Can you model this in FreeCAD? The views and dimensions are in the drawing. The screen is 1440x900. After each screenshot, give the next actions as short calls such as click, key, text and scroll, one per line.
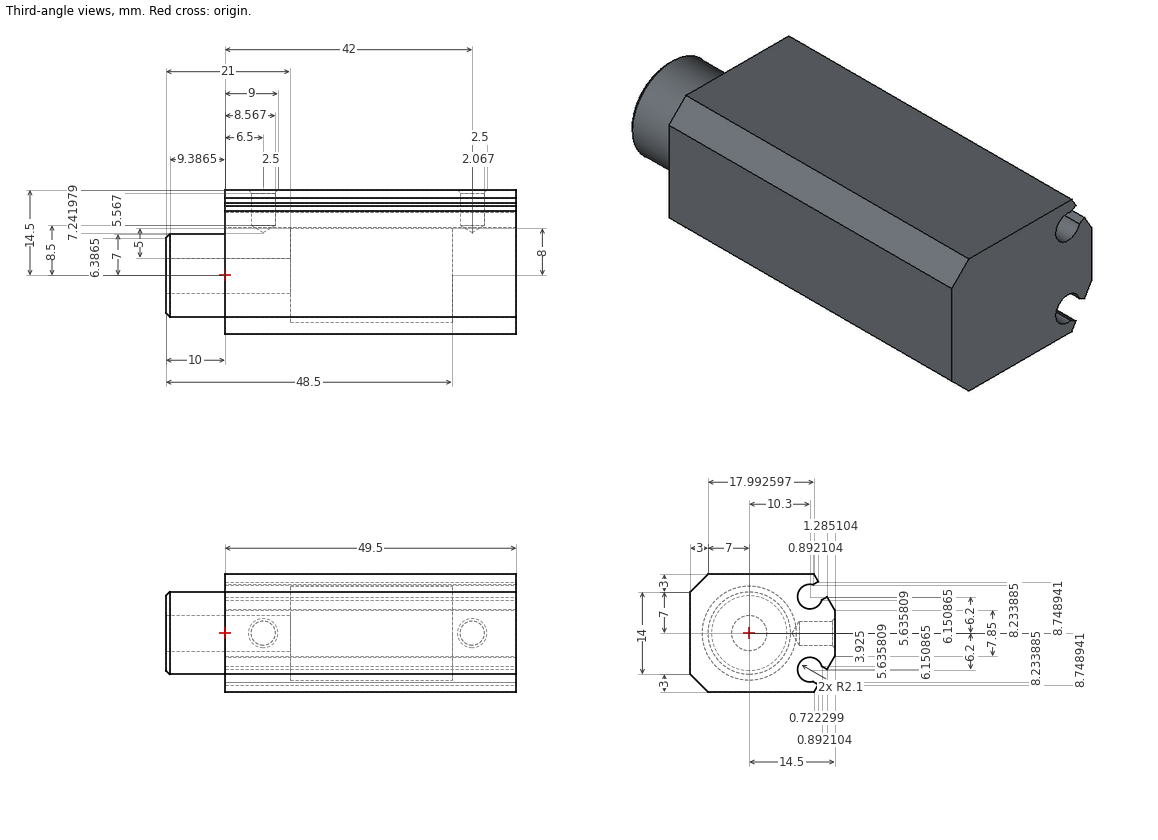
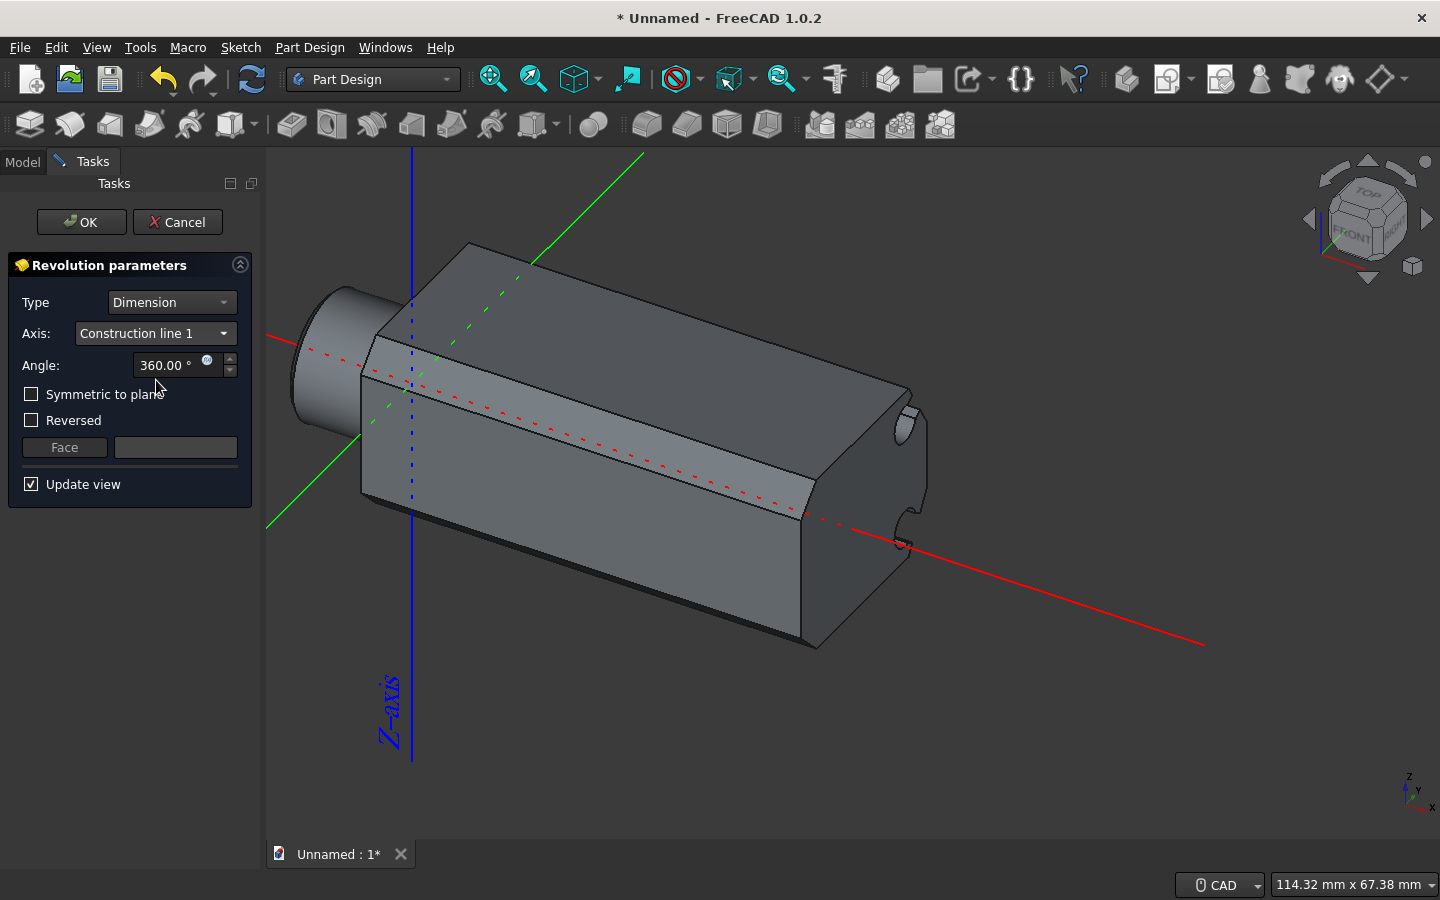
click(82, 222)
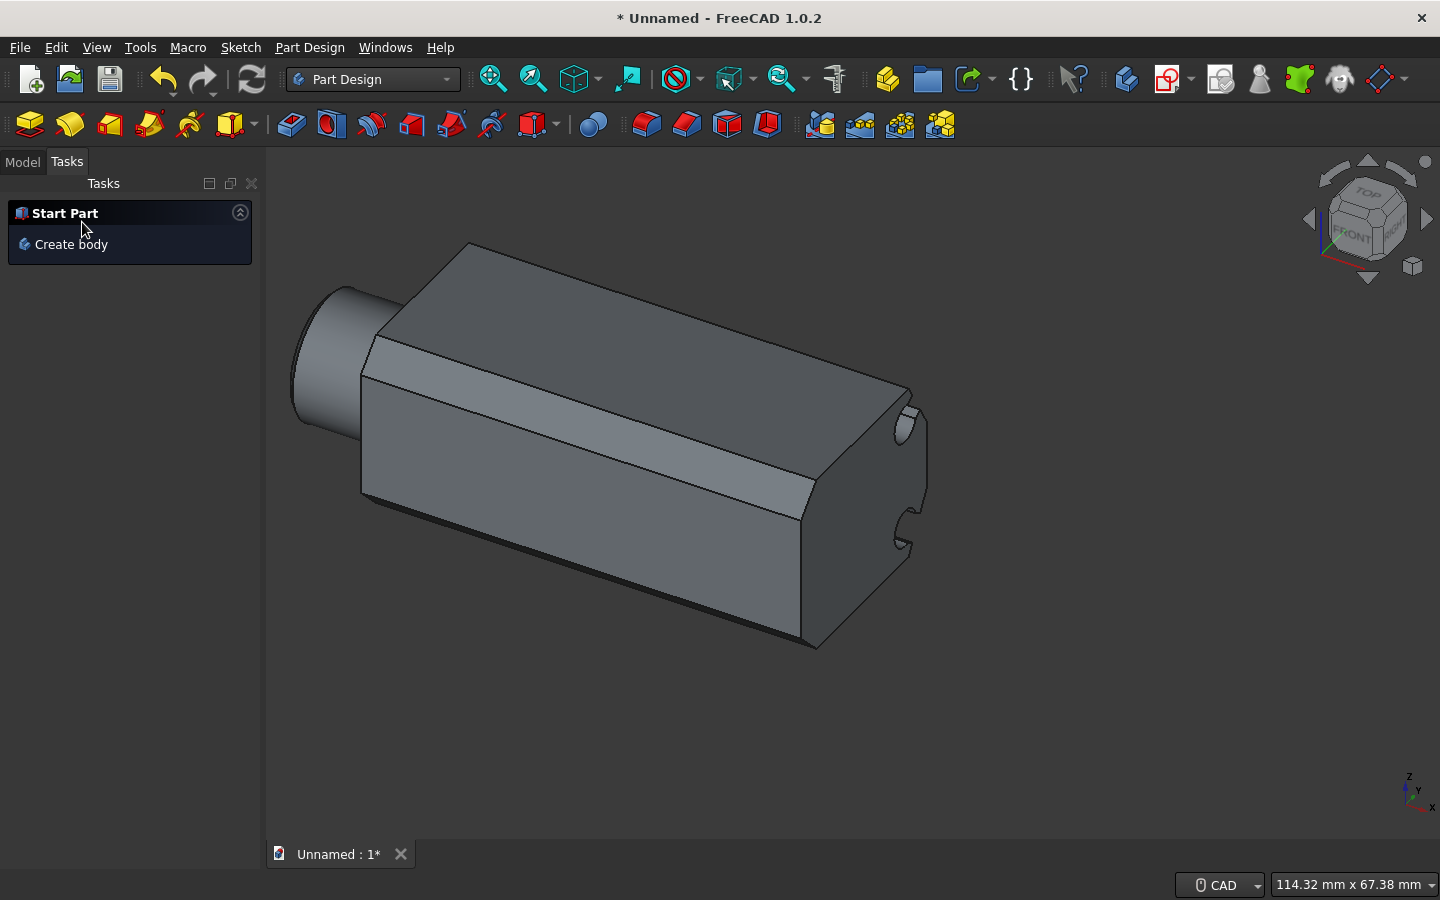
click(1168, 80)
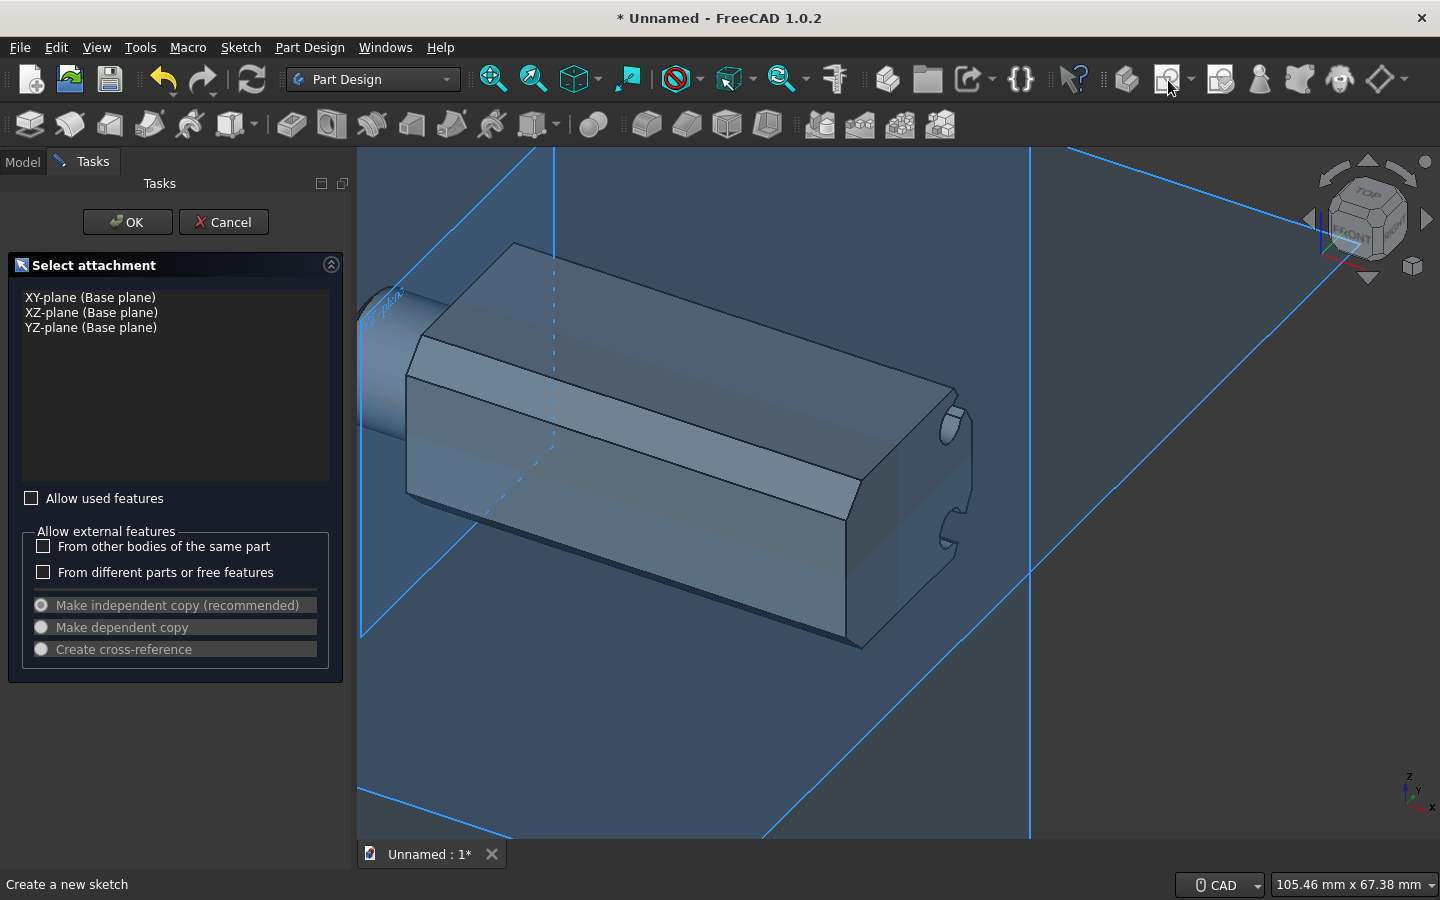
click(82, 298)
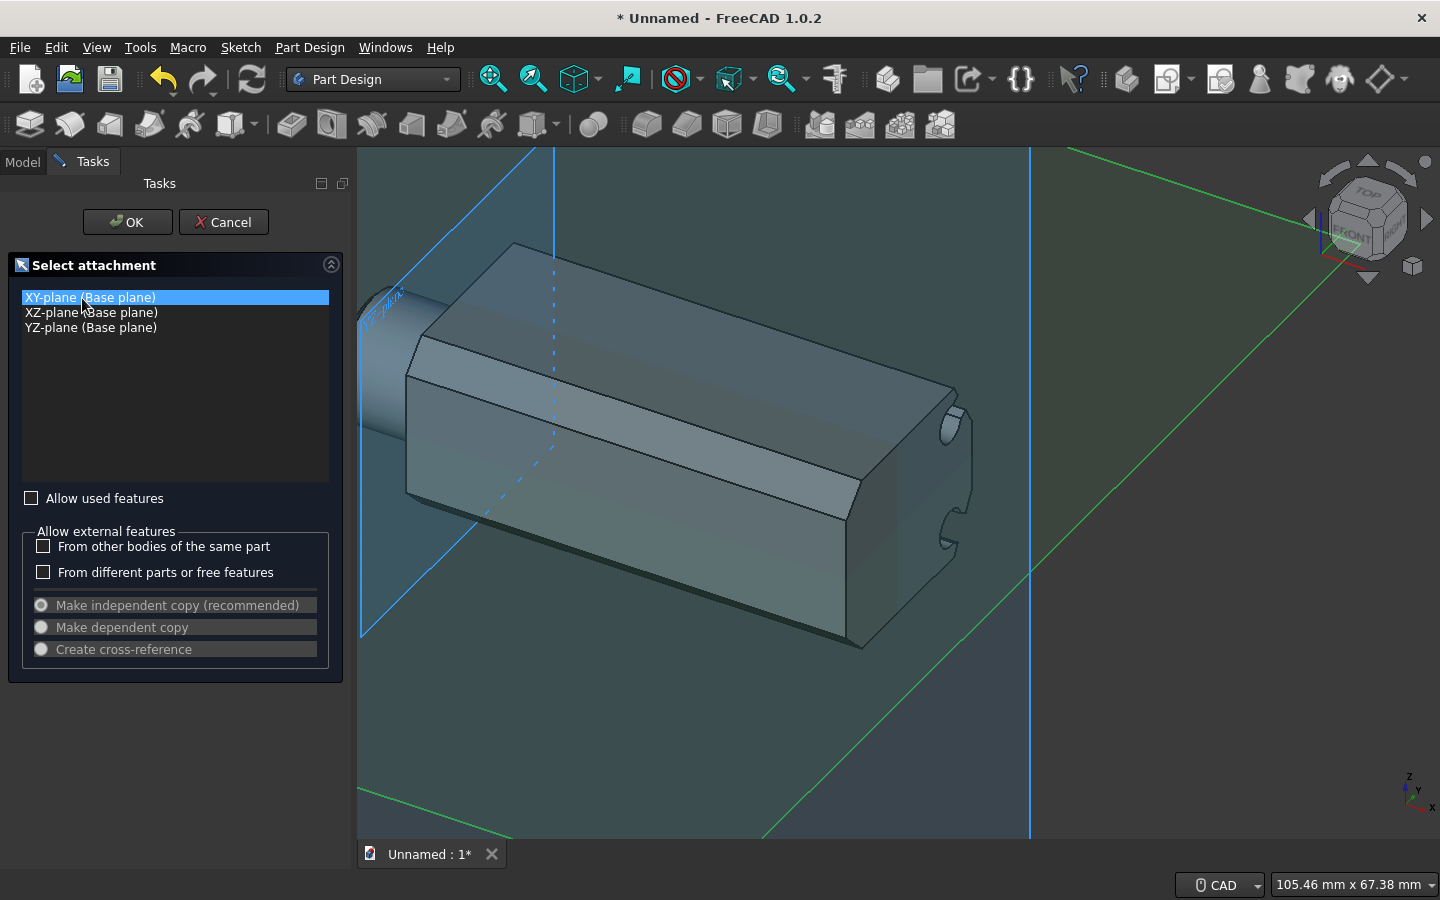
click(128, 222)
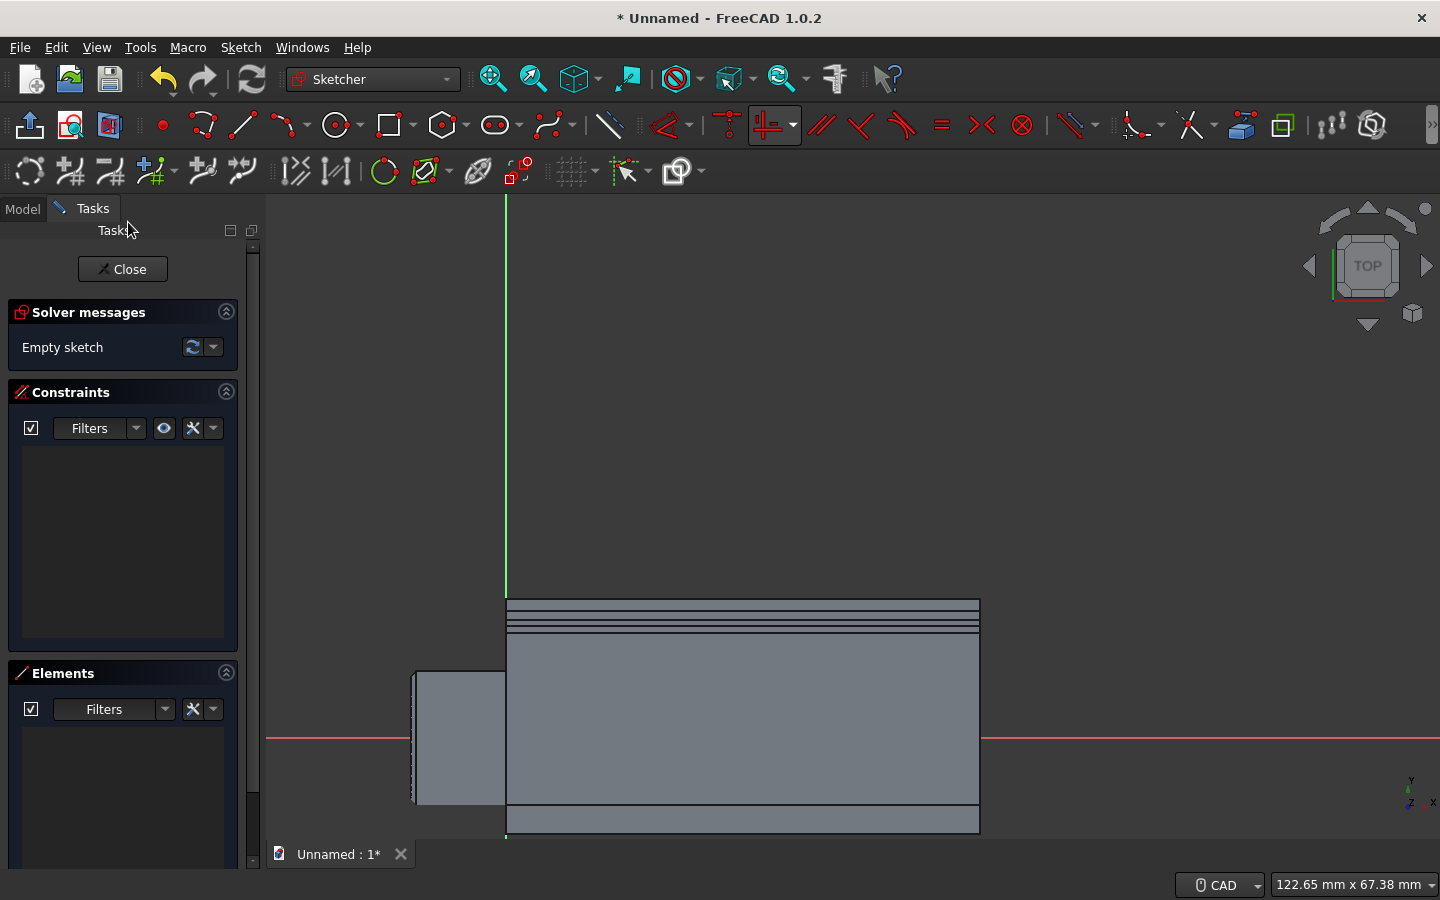
click(110, 126)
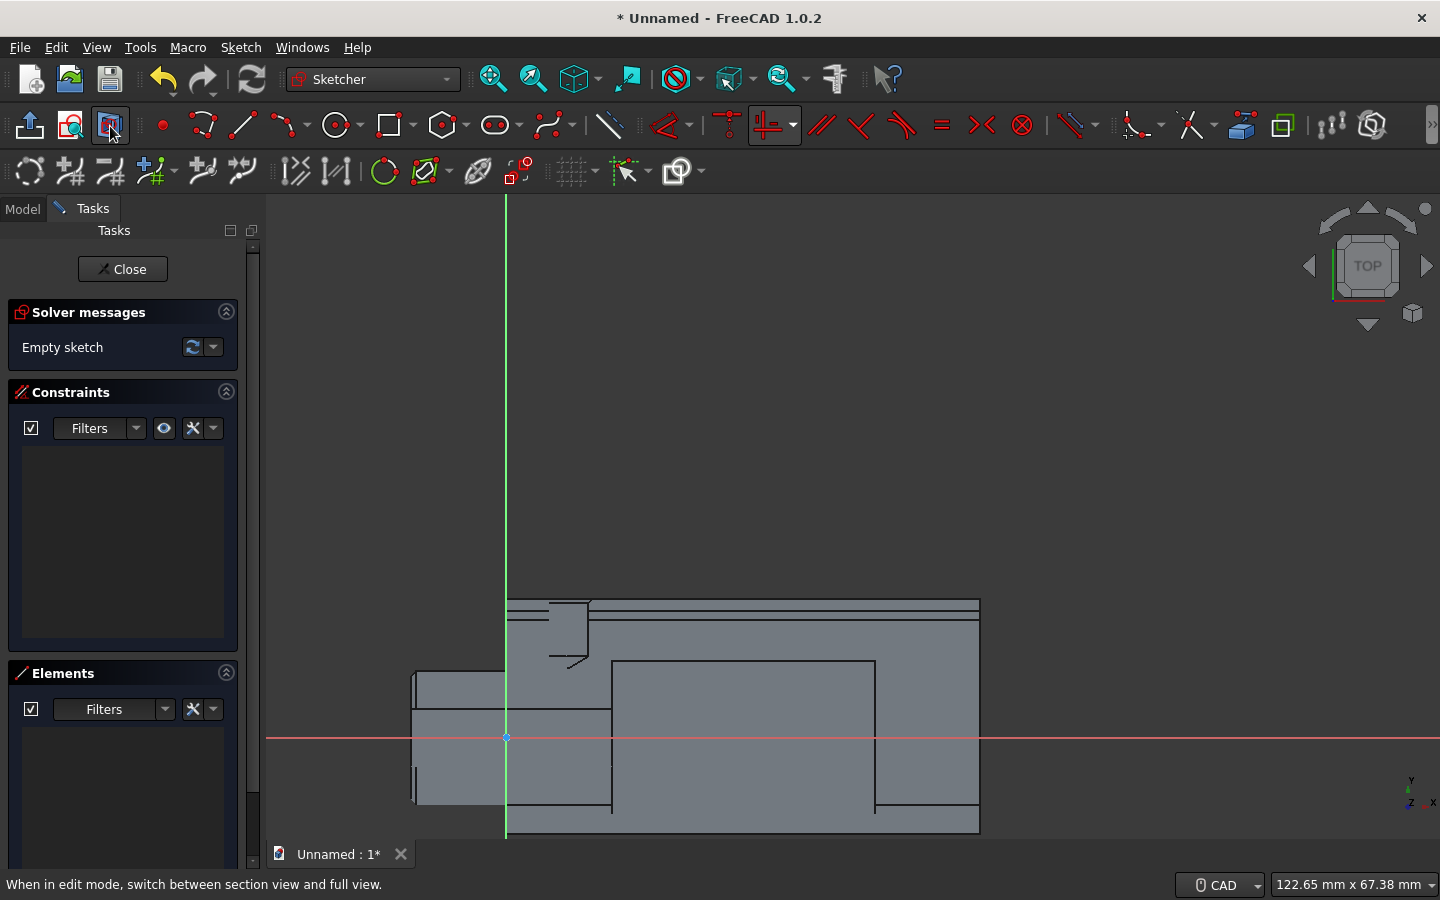
scroll(965, 654, up, 7)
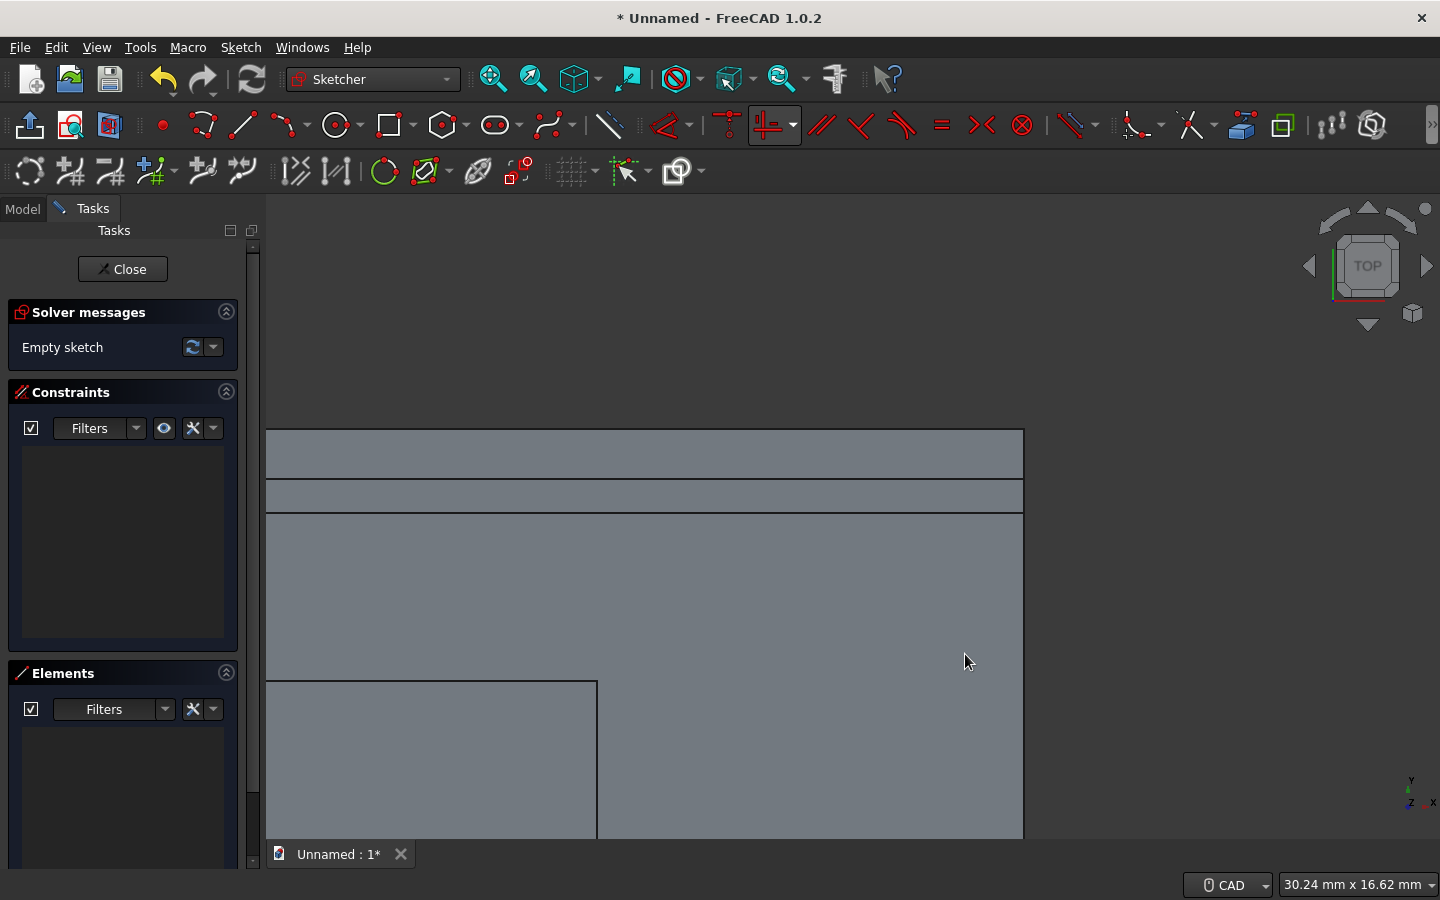
key(g)
key(m)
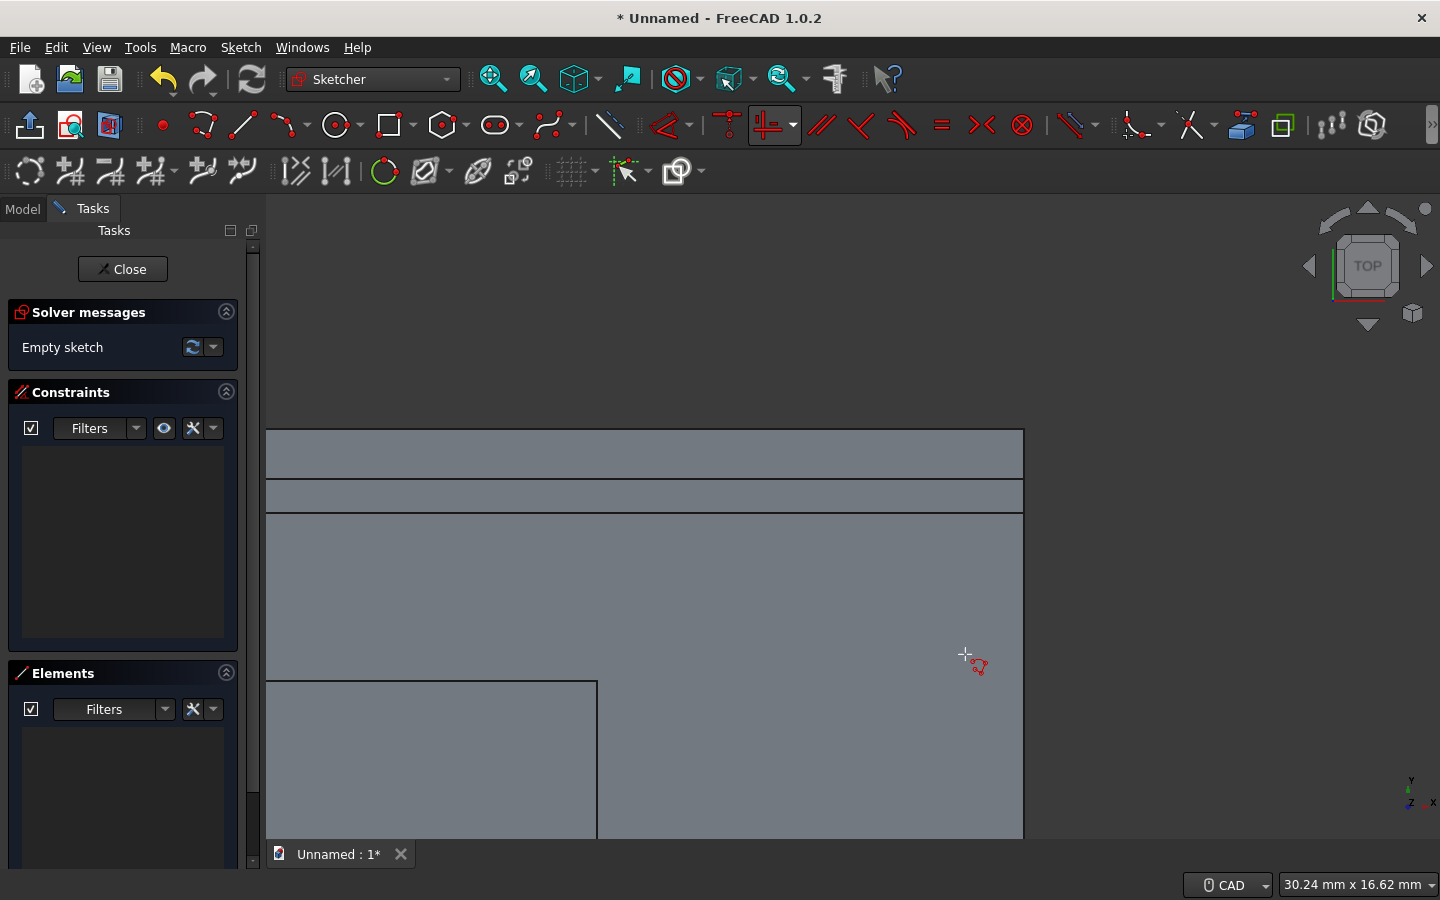
click(733, 710)
click(813, 662)
click(813, 446)
click(830, 429)
click(733, 429)
click(733, 711)